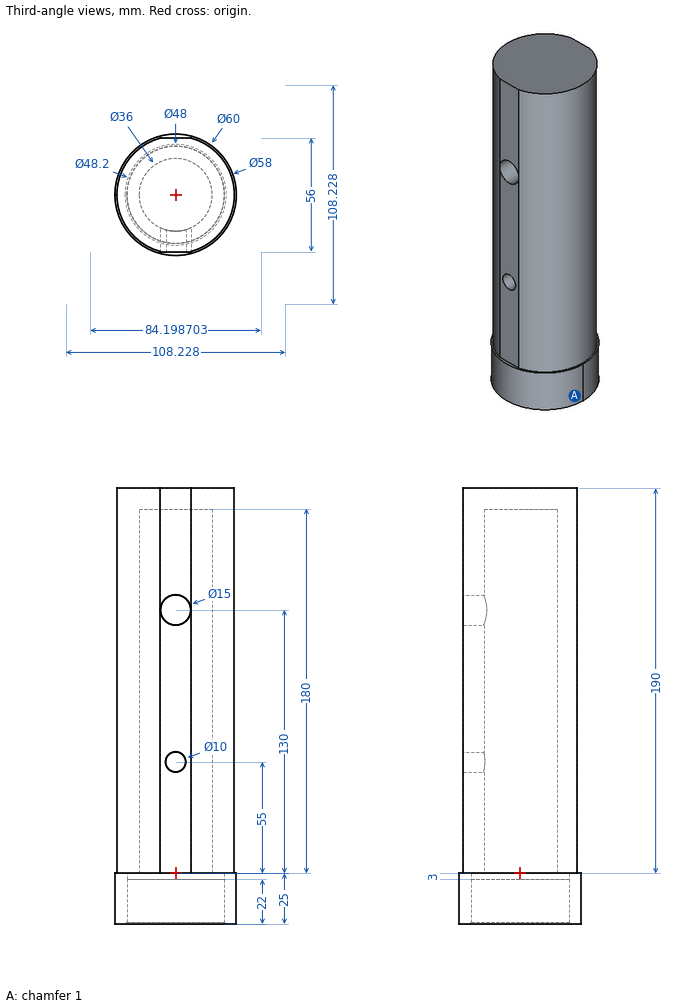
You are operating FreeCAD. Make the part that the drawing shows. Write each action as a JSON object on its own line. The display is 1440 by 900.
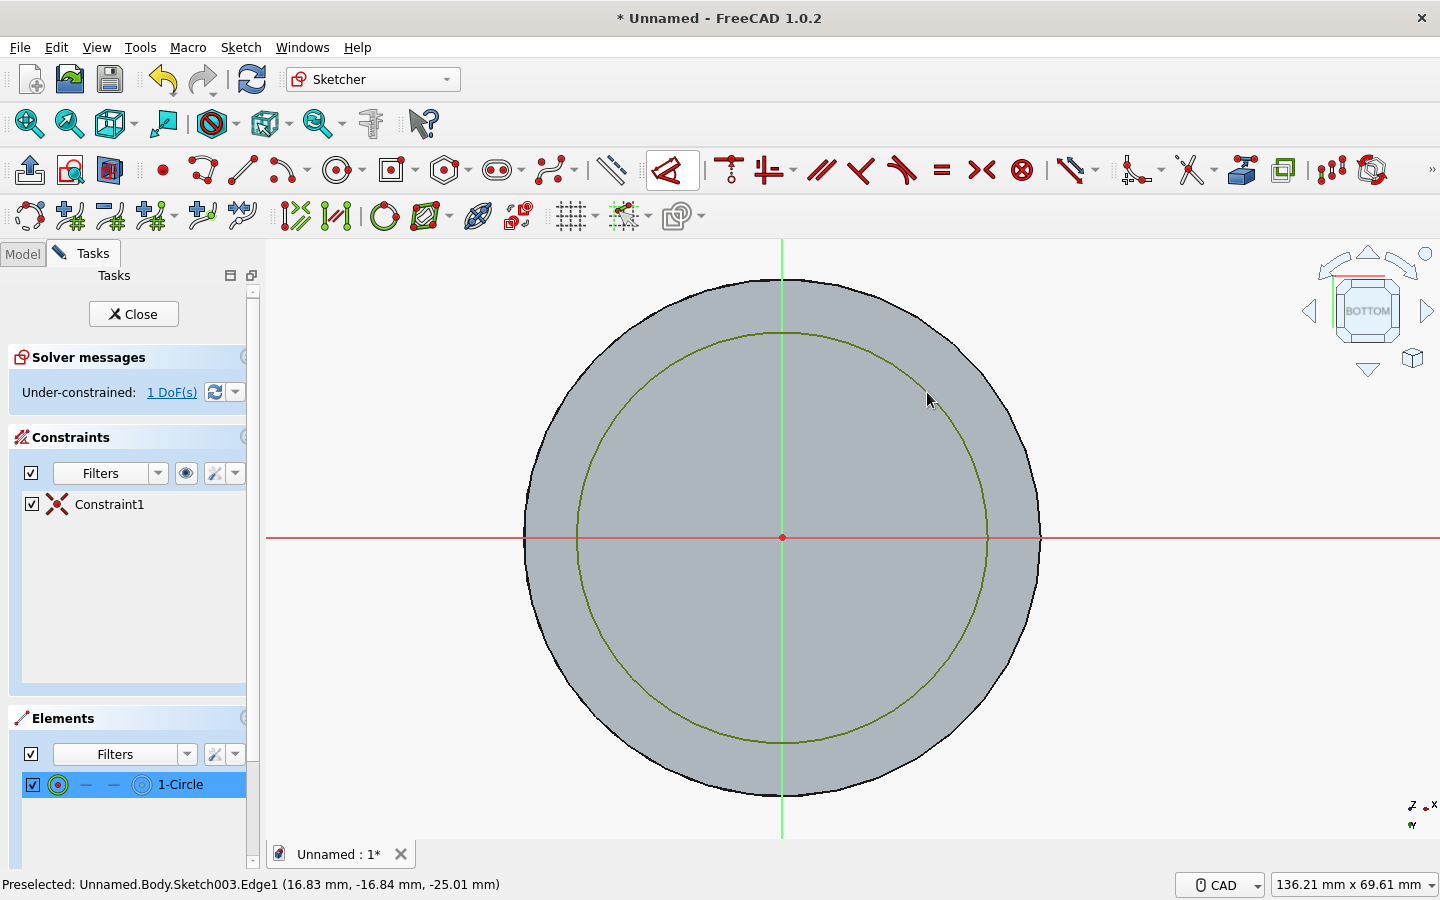
{"action": "left_click", "coordinate": [694, 170]}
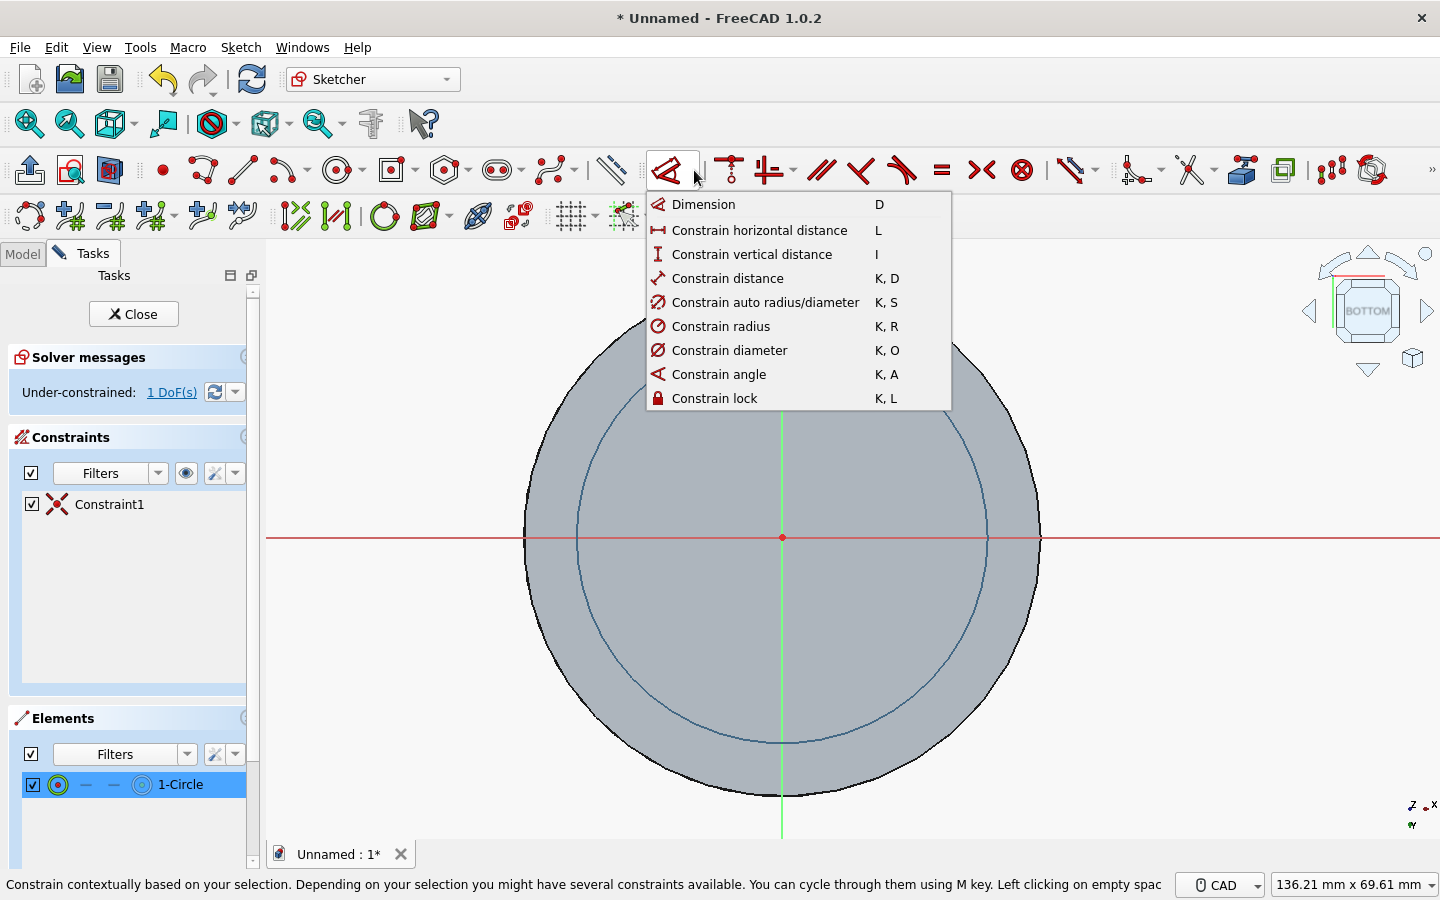
{"action": "left_click", "coordinate": [799, 350]}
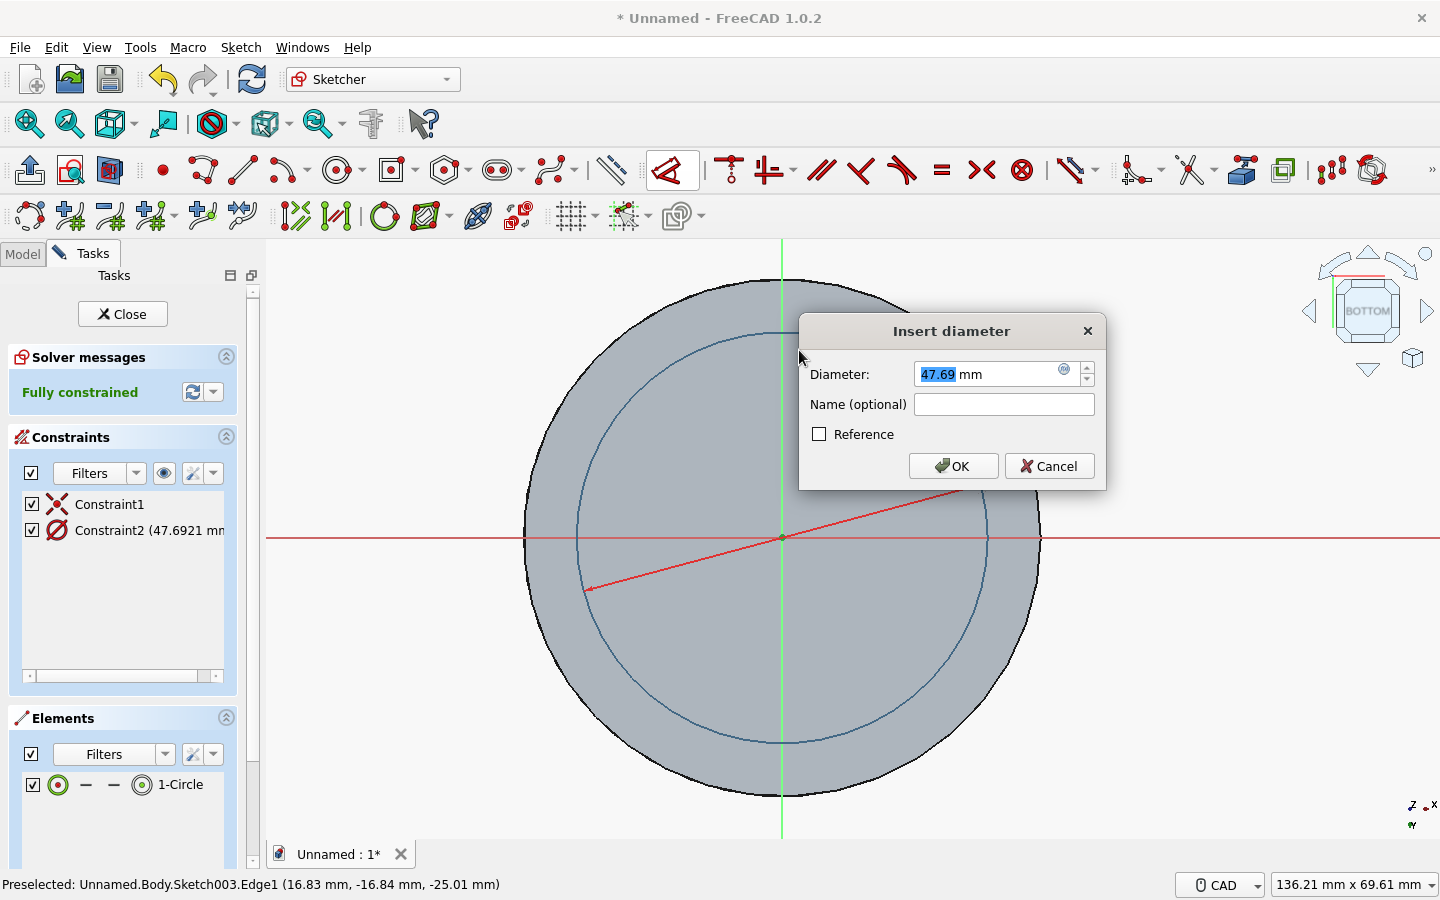
{"action": "type", "text": "48"}
{"action": "key", "text": "Return"}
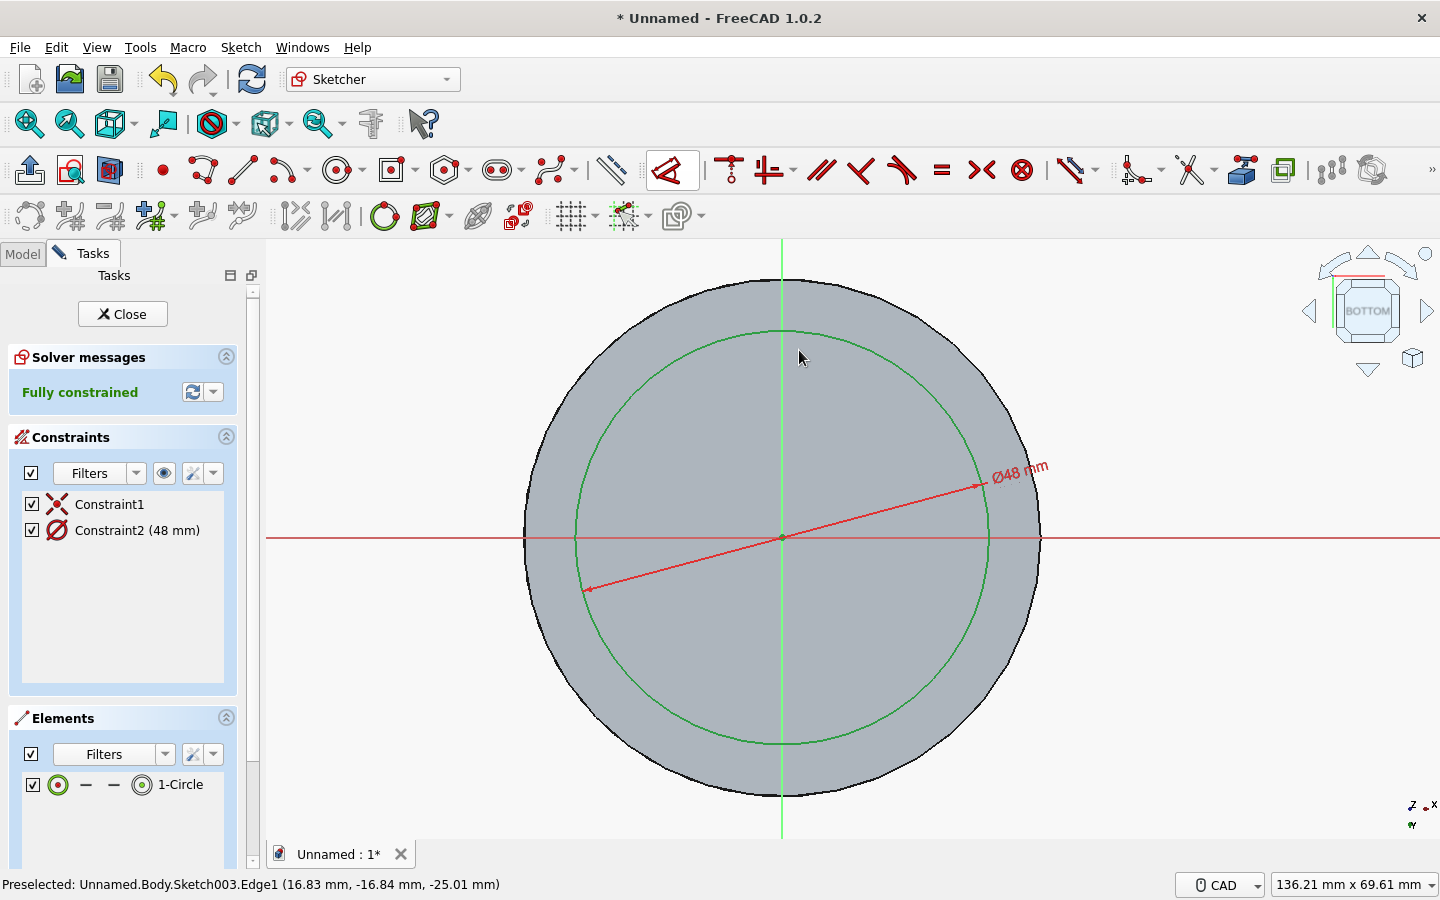
{"action": "left_click", "coordinate": [123, 314]}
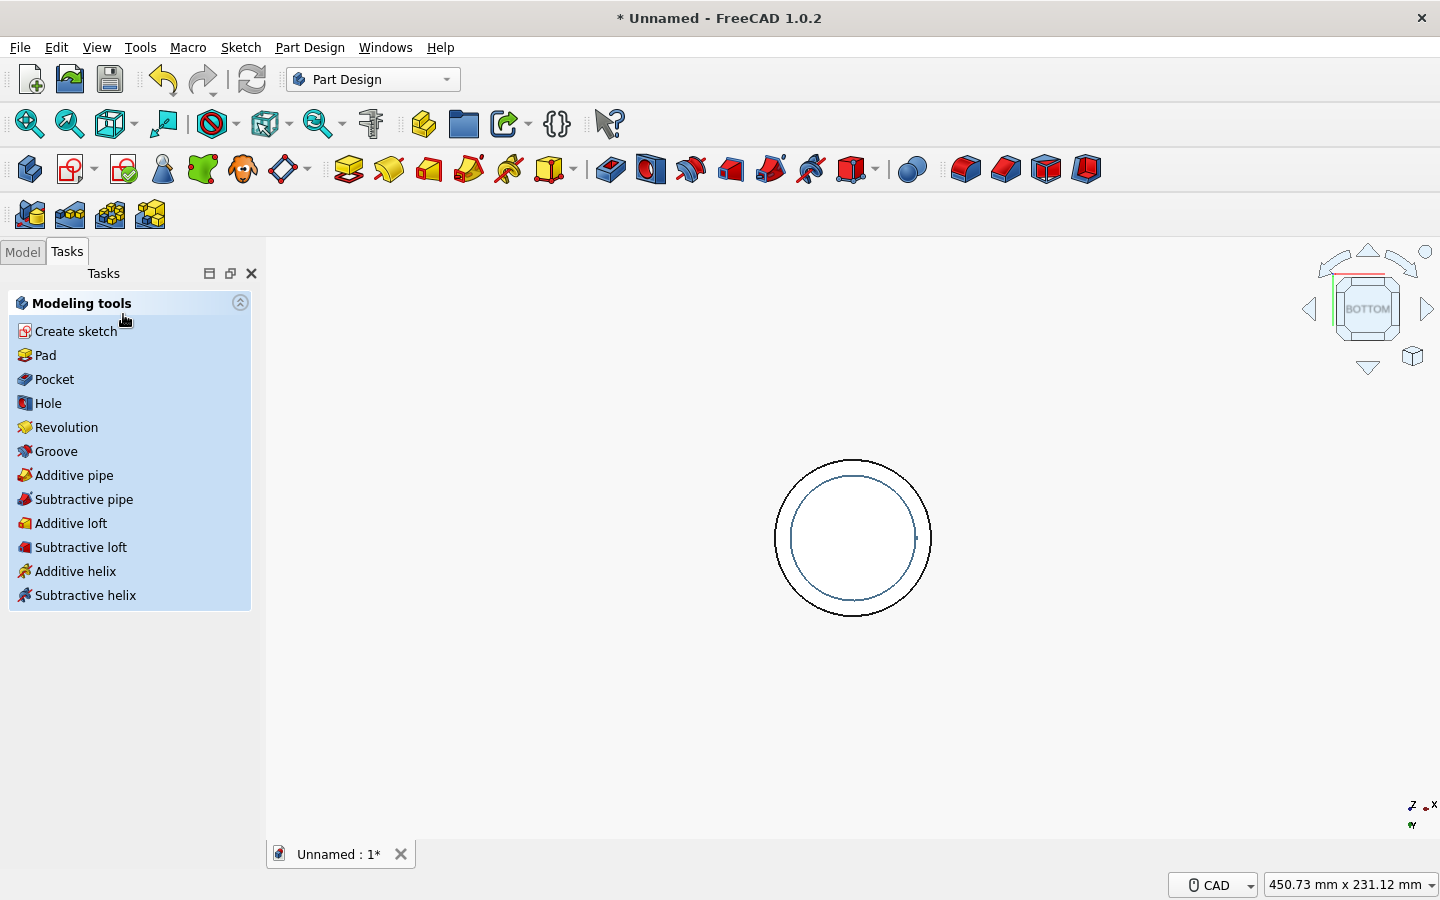
{"action": "left_click", "coordinate": [612, 170]}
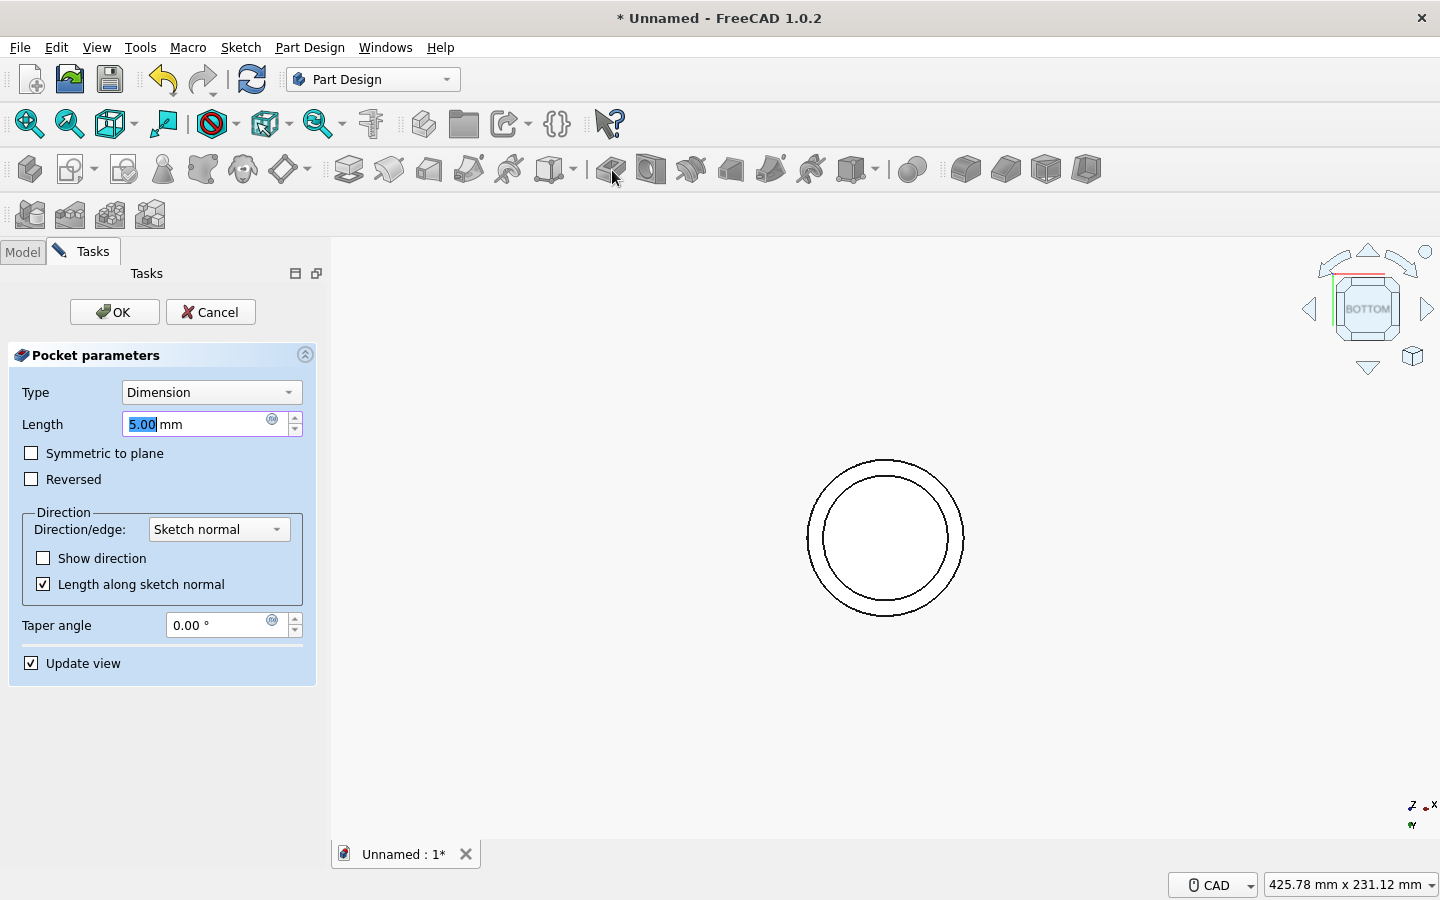
{"action": "type", "text": "22"}
{"action": "key", "text": "Tab"}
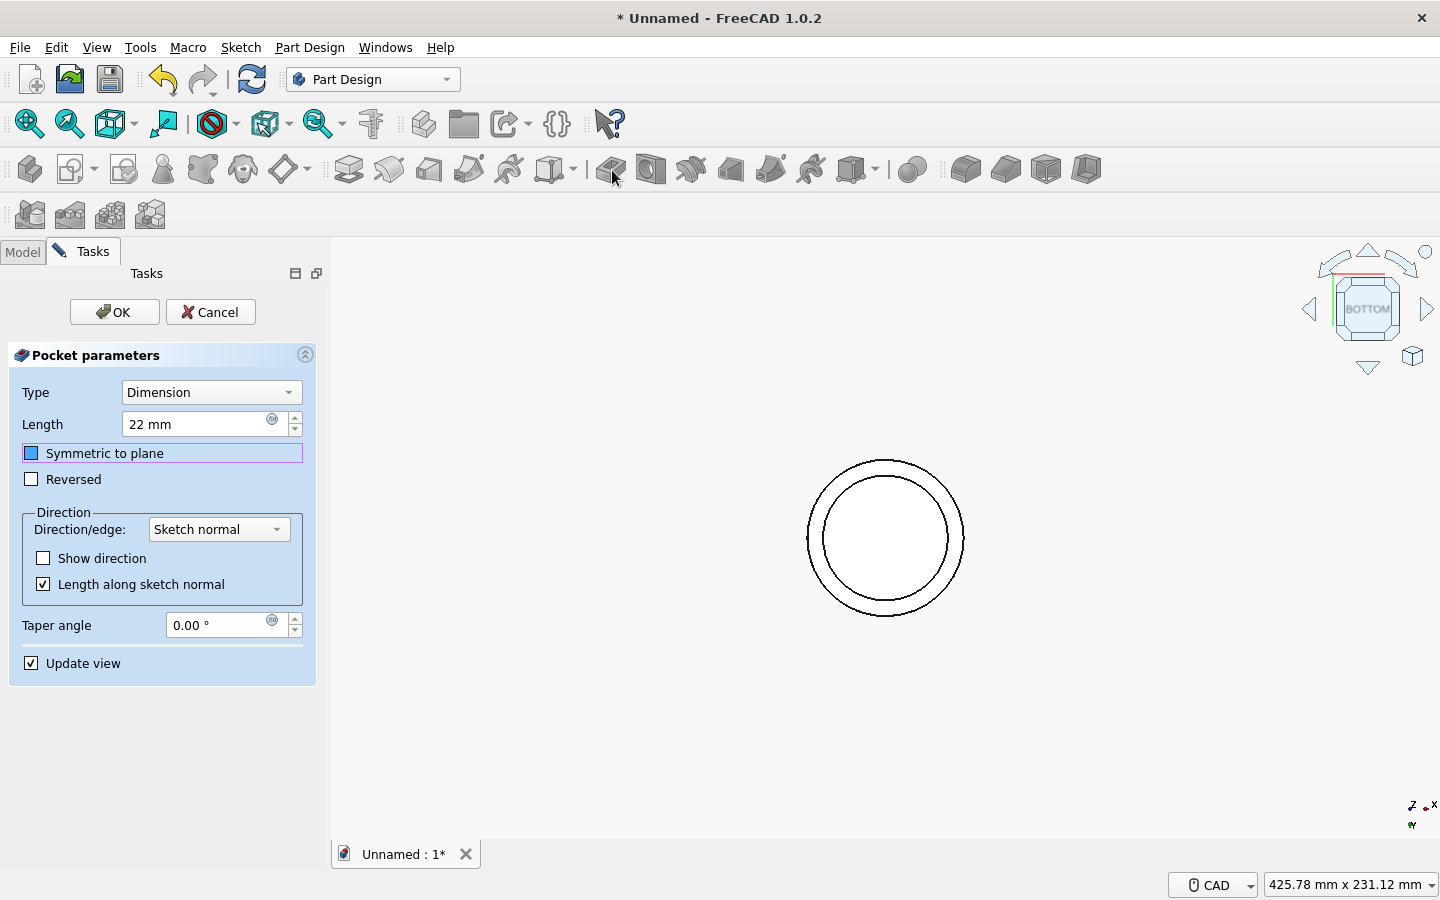
{"action": "left_click", "coordinate": [115, 312]}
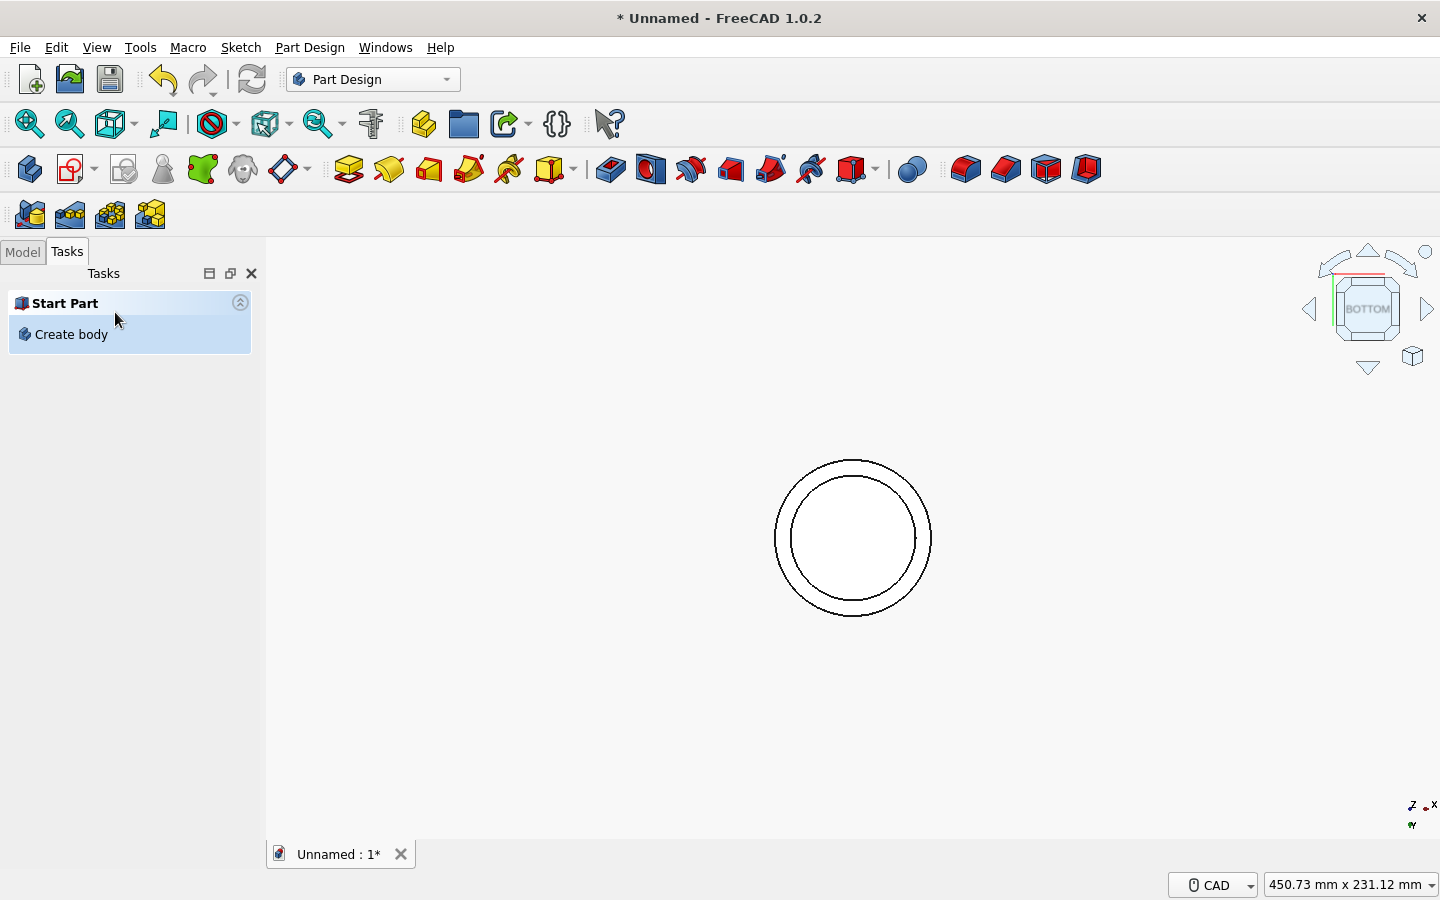
{"action": "left_click", "coordinate": [30, 124]}